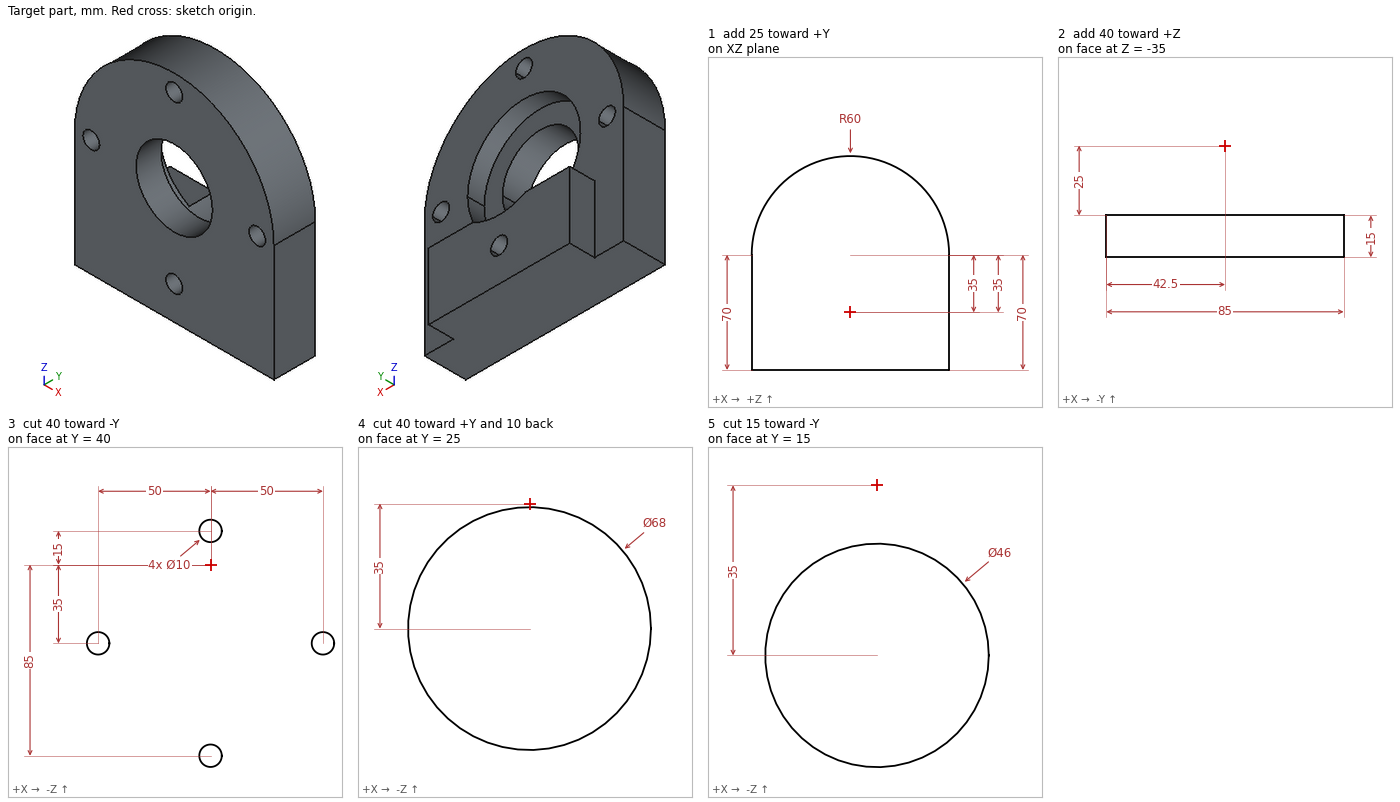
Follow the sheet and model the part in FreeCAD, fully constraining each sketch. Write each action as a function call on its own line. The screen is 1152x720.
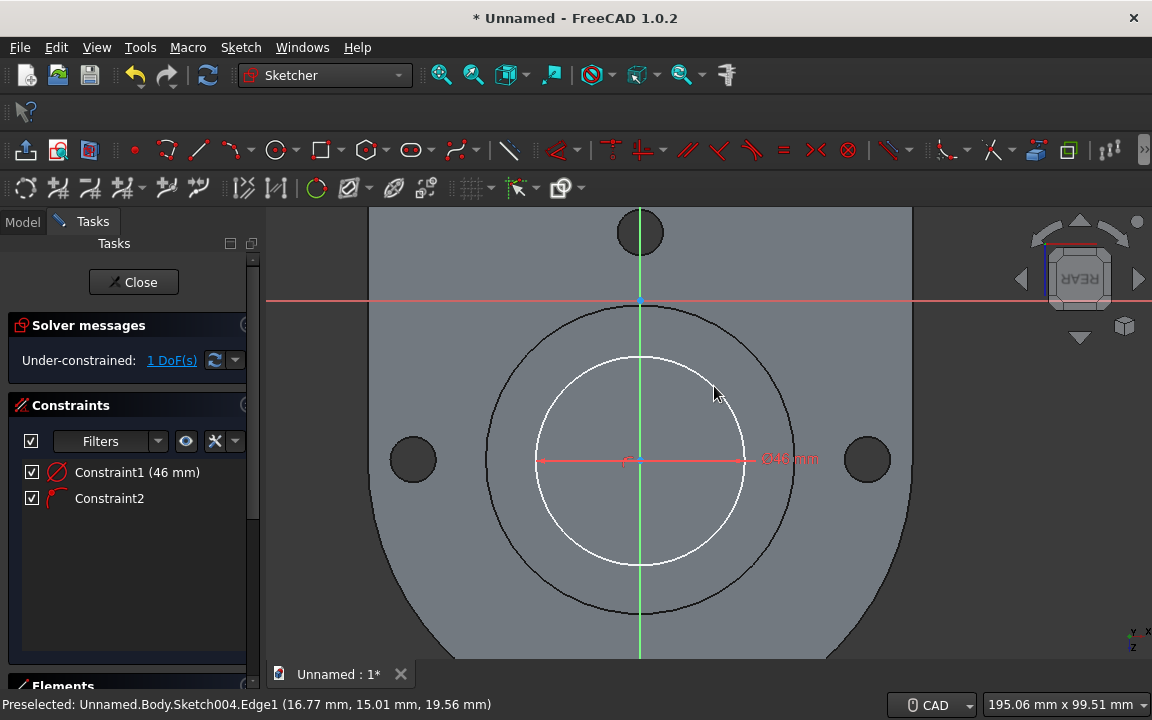
key(d)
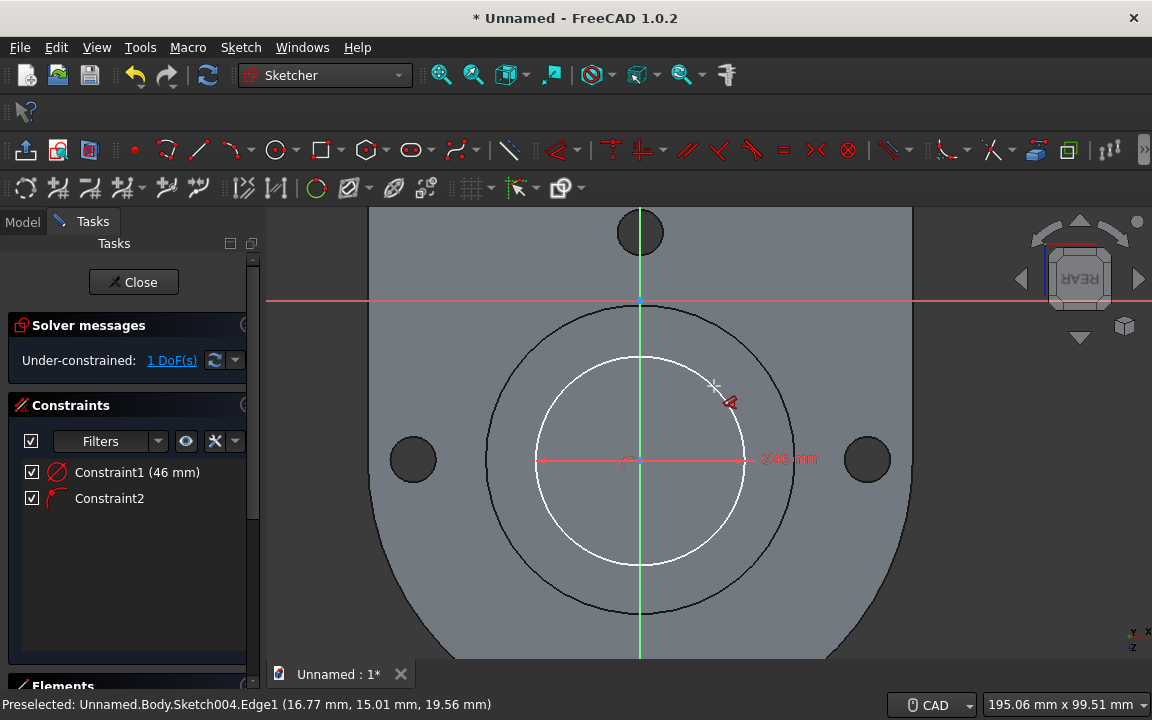
click(640, 461)
click(674, 381)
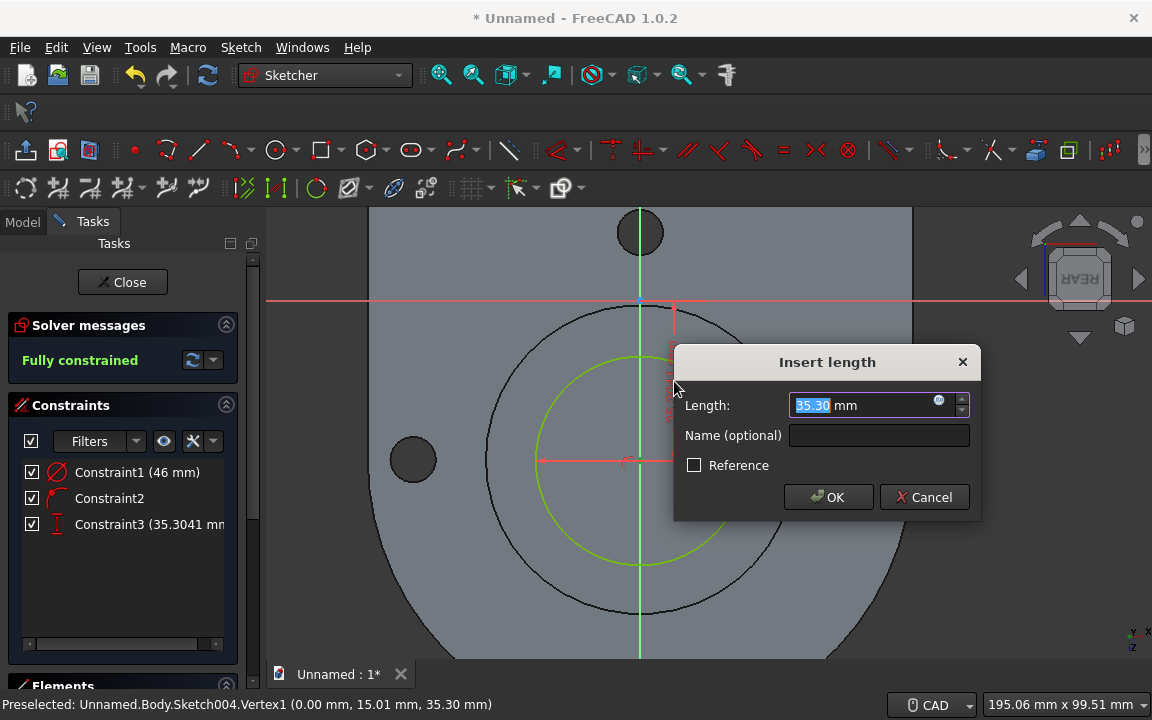
text(35)
key(Return)
key(Escape)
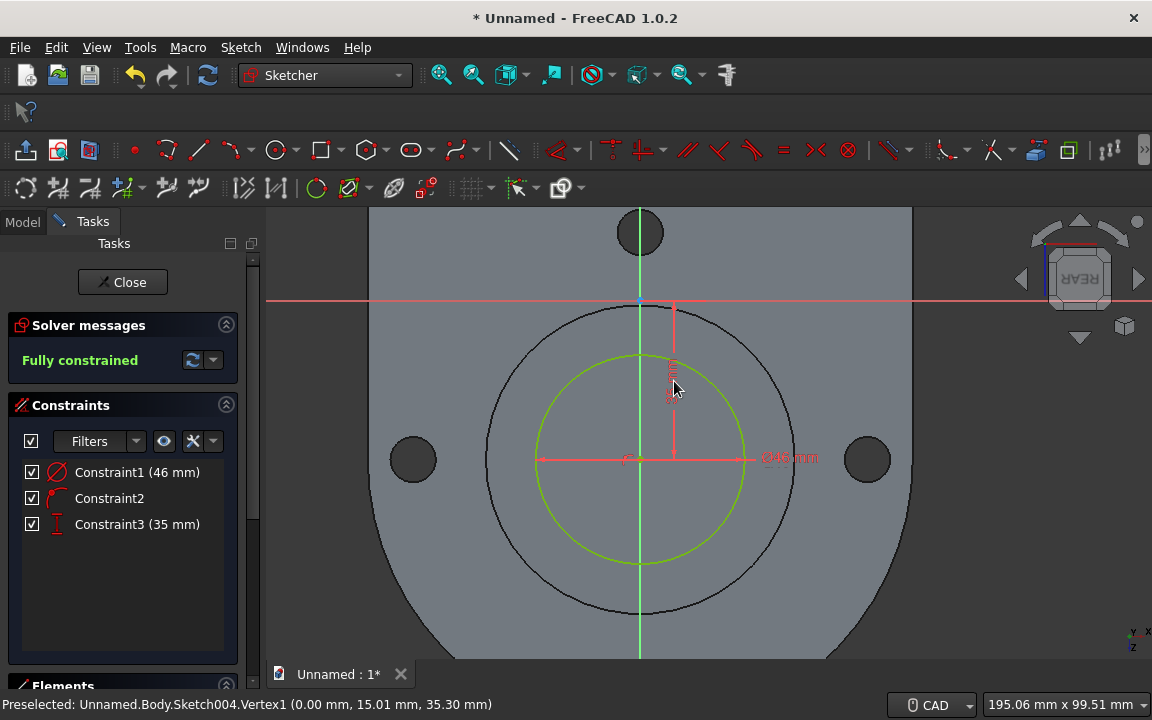
click(123, 282)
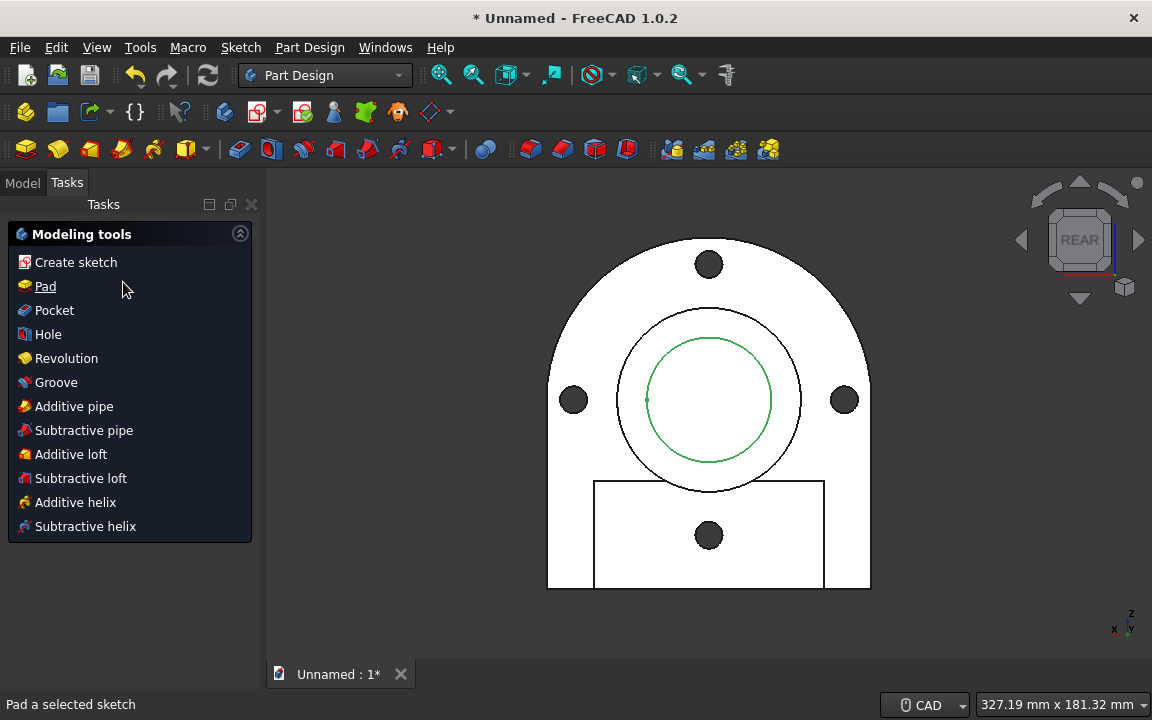
click(240, 150)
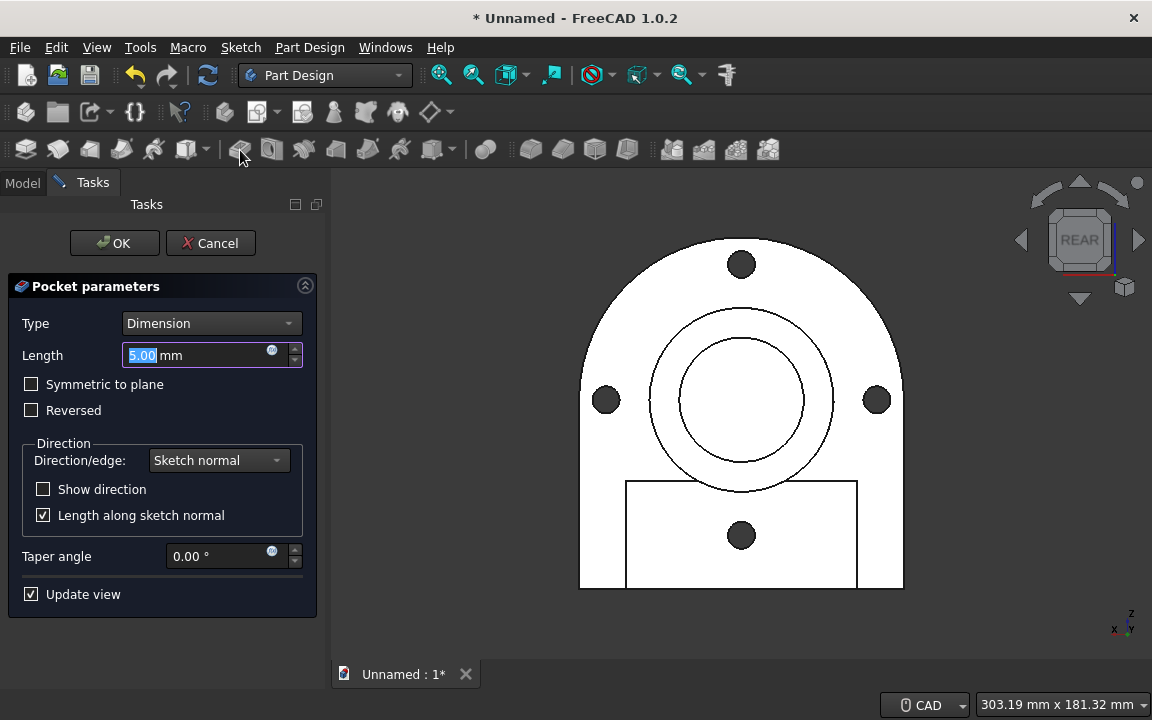
text(15)
key(Tab)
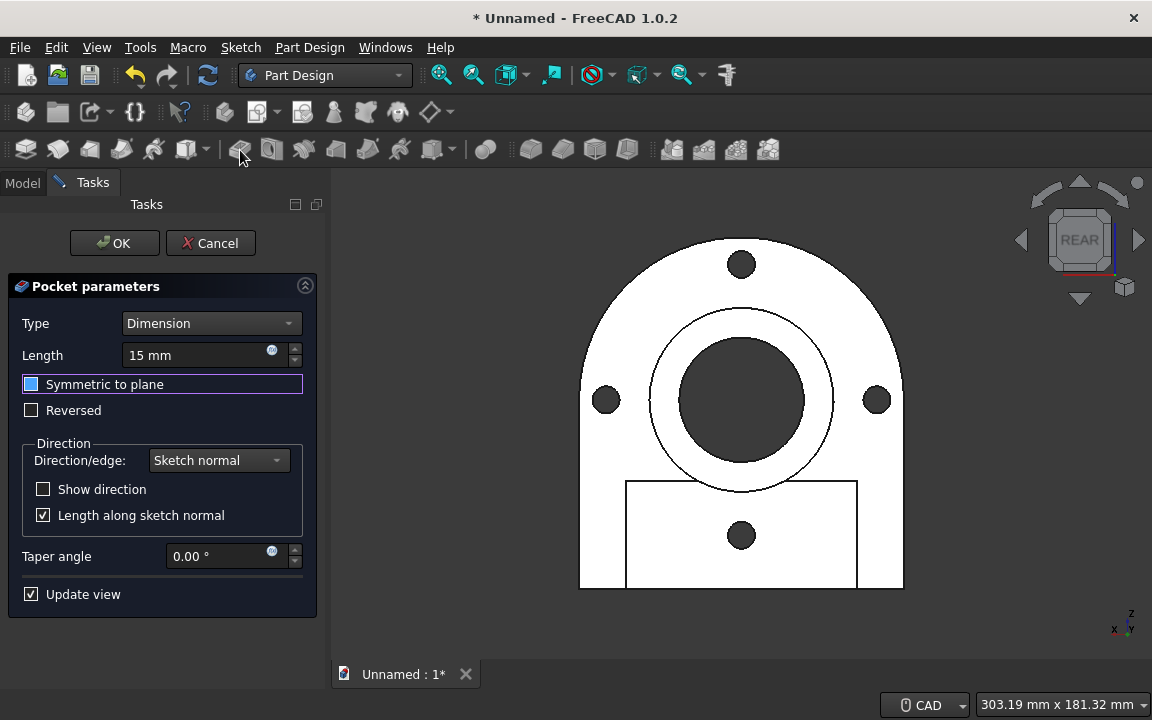
click(115, 243)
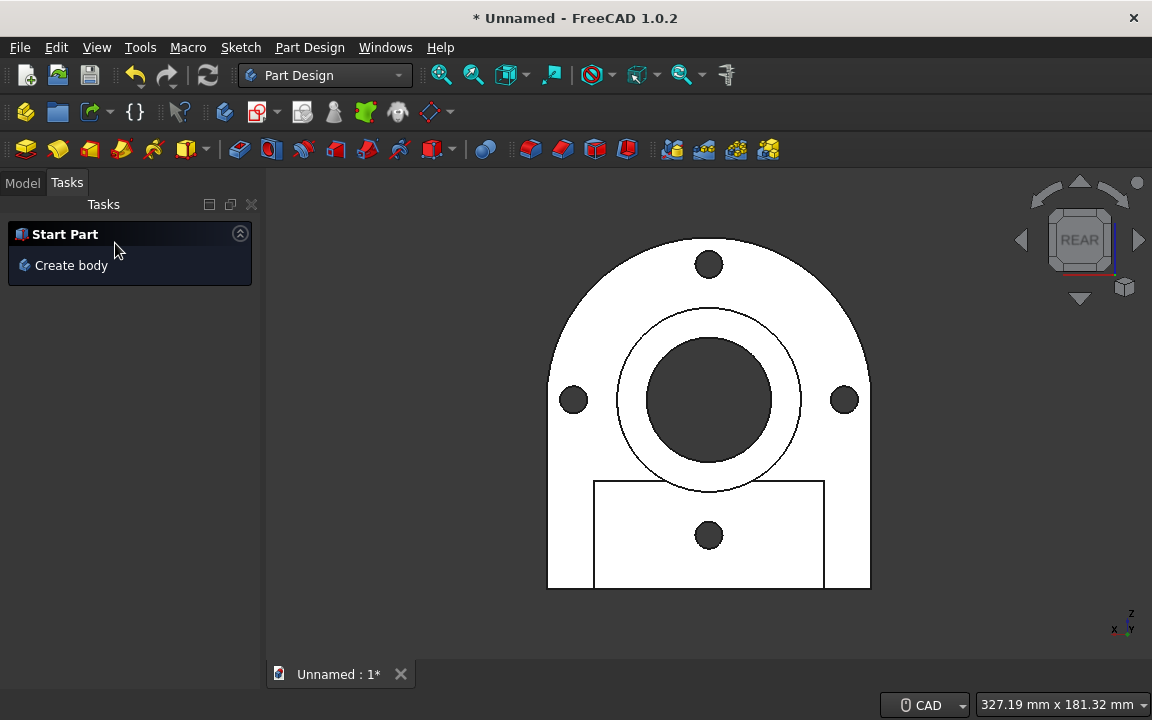
key(0)